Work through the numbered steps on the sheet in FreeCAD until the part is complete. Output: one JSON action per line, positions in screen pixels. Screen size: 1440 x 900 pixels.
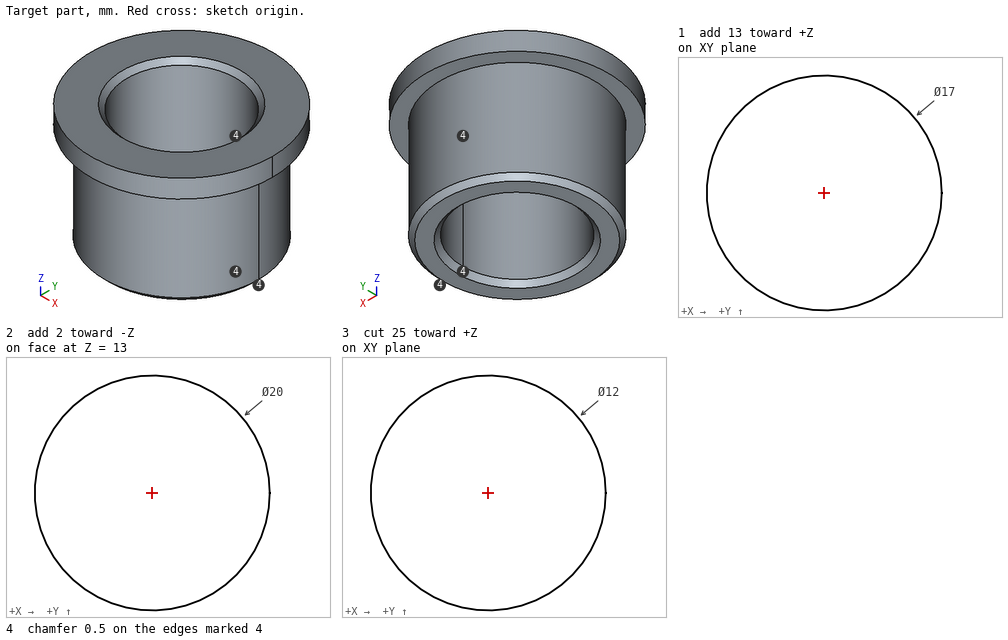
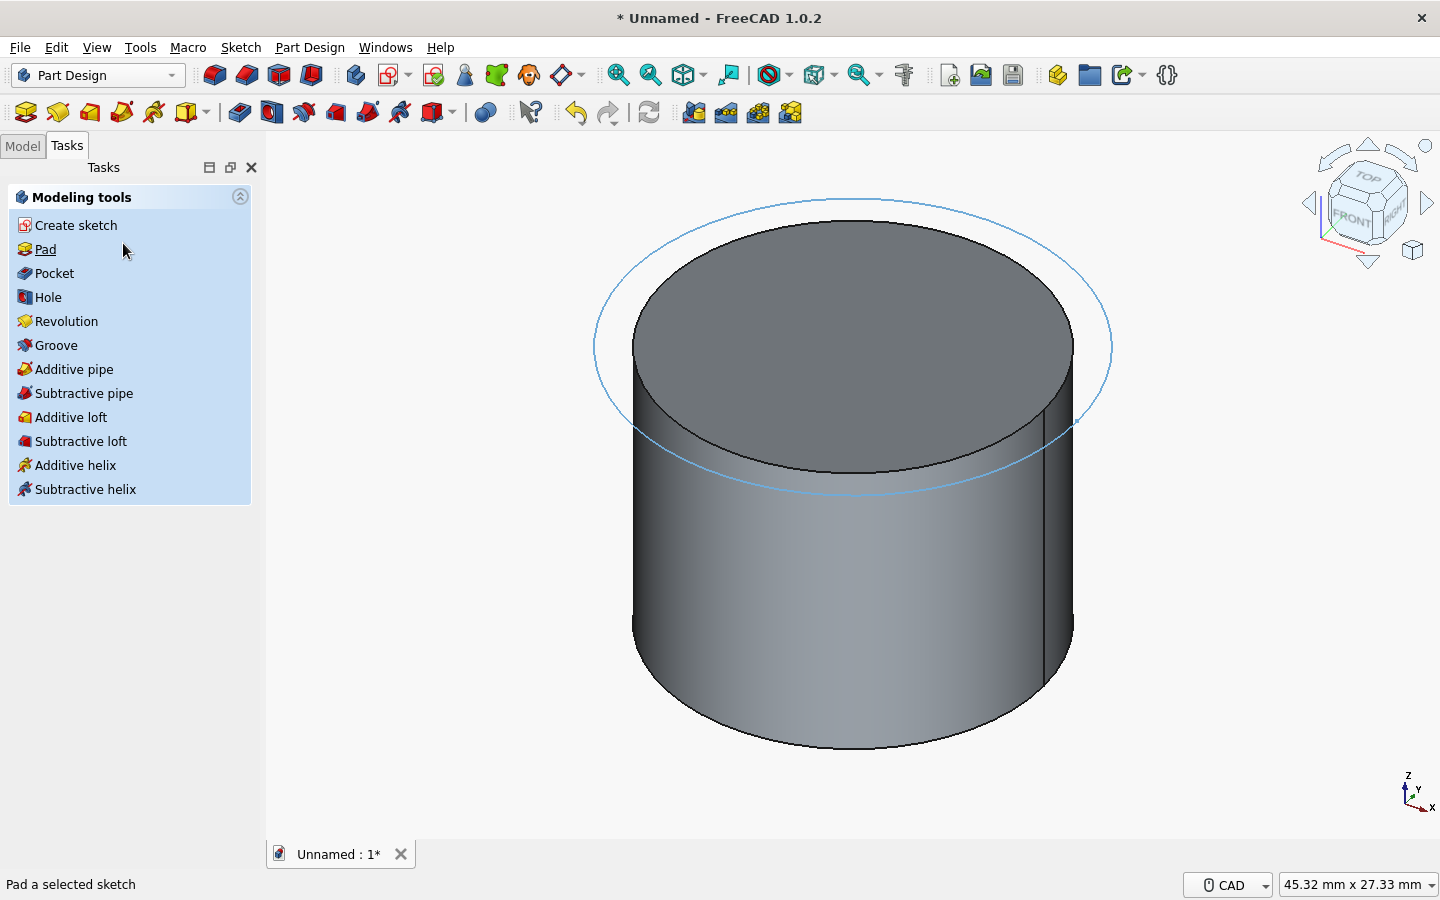
{"action": "left_click", "coordinate": [26, 112]}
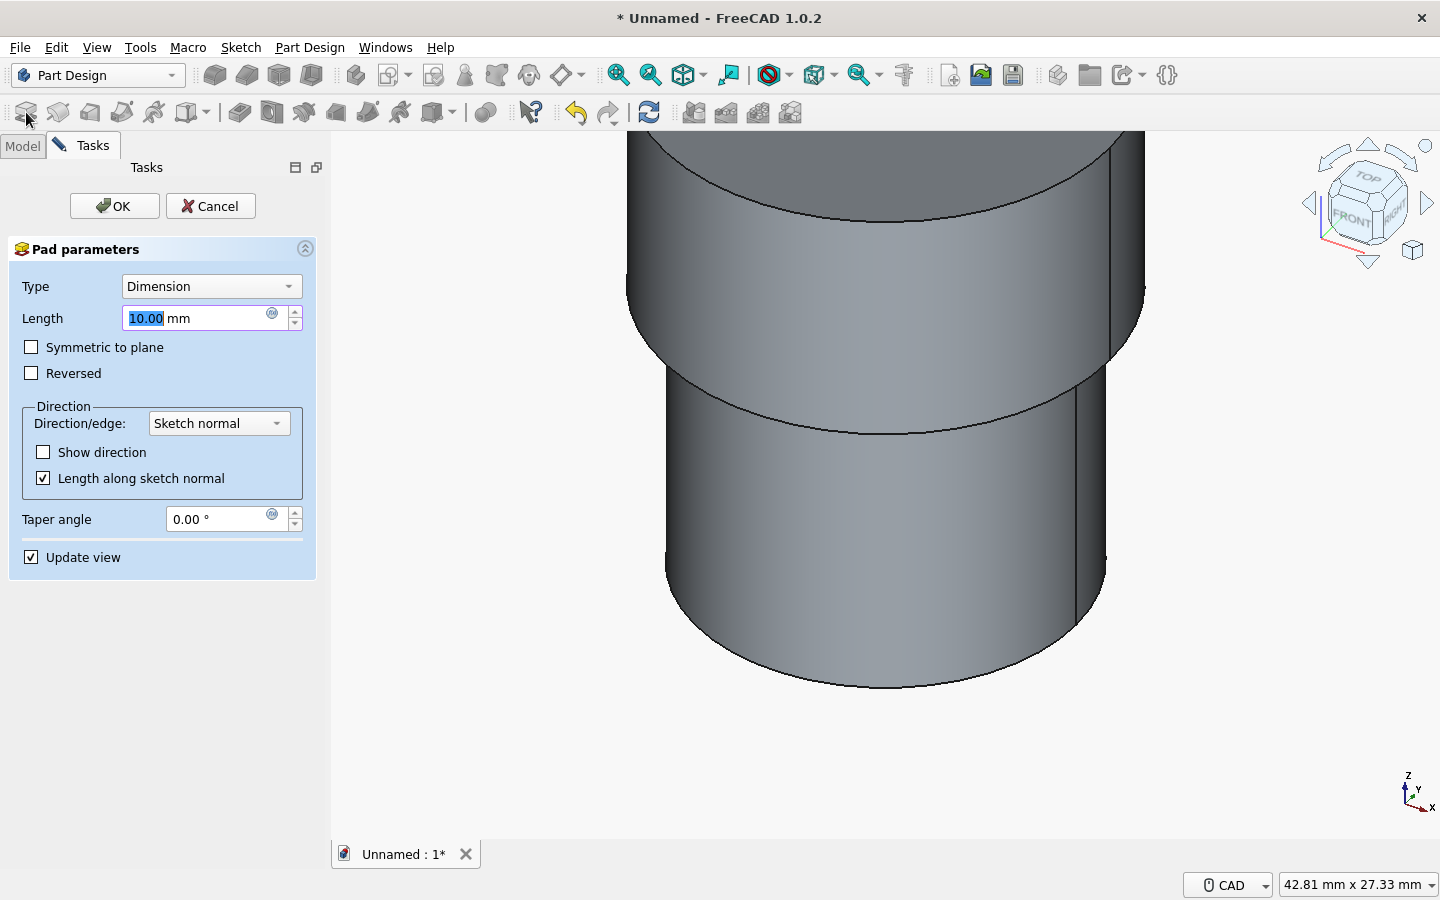
{"action": "type", "text": "2"}
{"action": "key", "text": "Tab"}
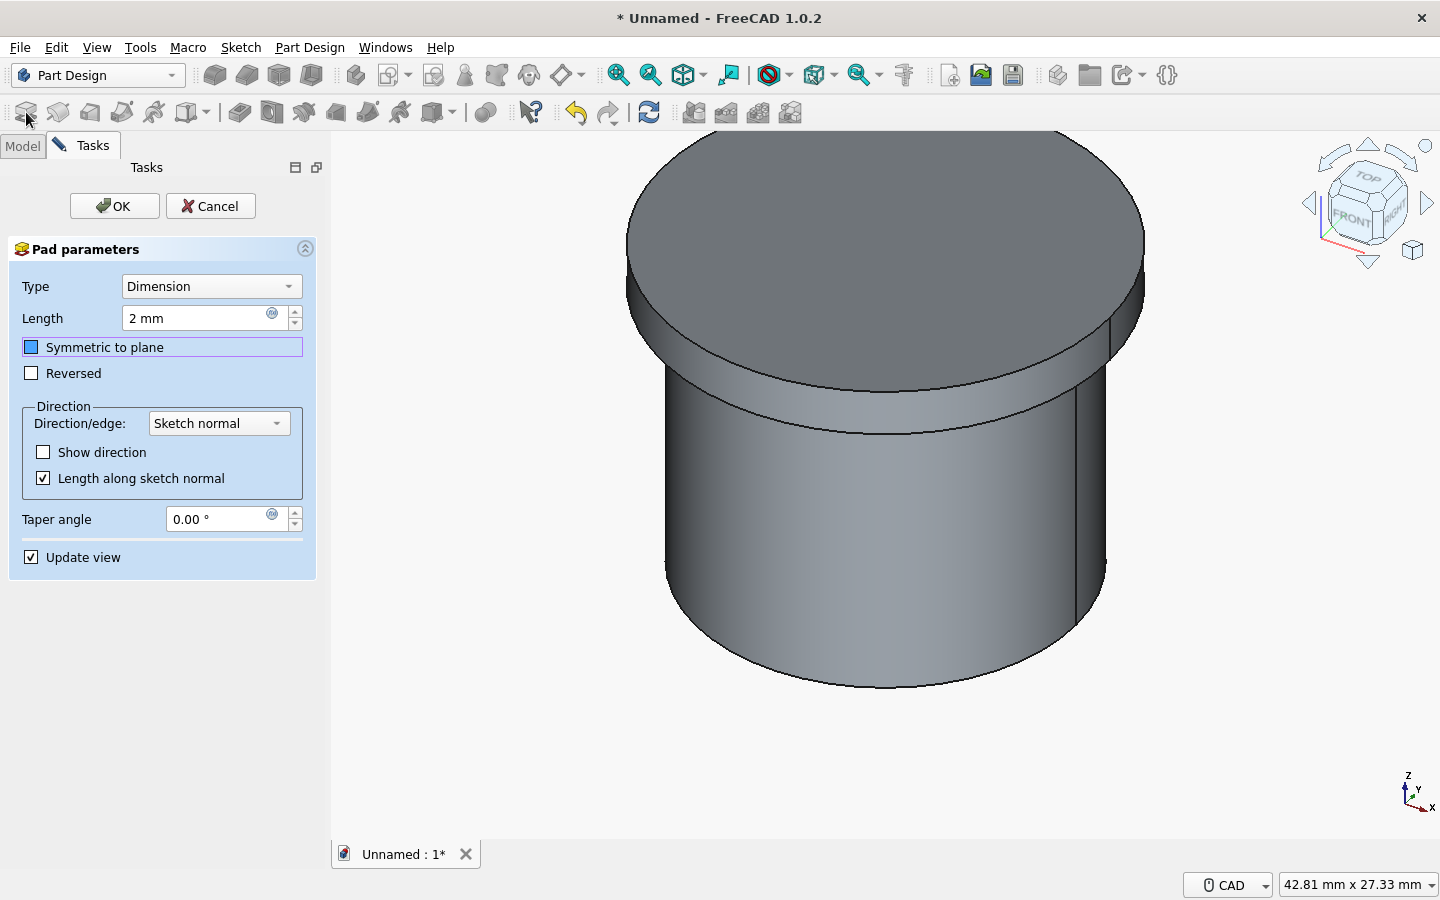
{"action": "left_click", "coordinate": [30, 373]}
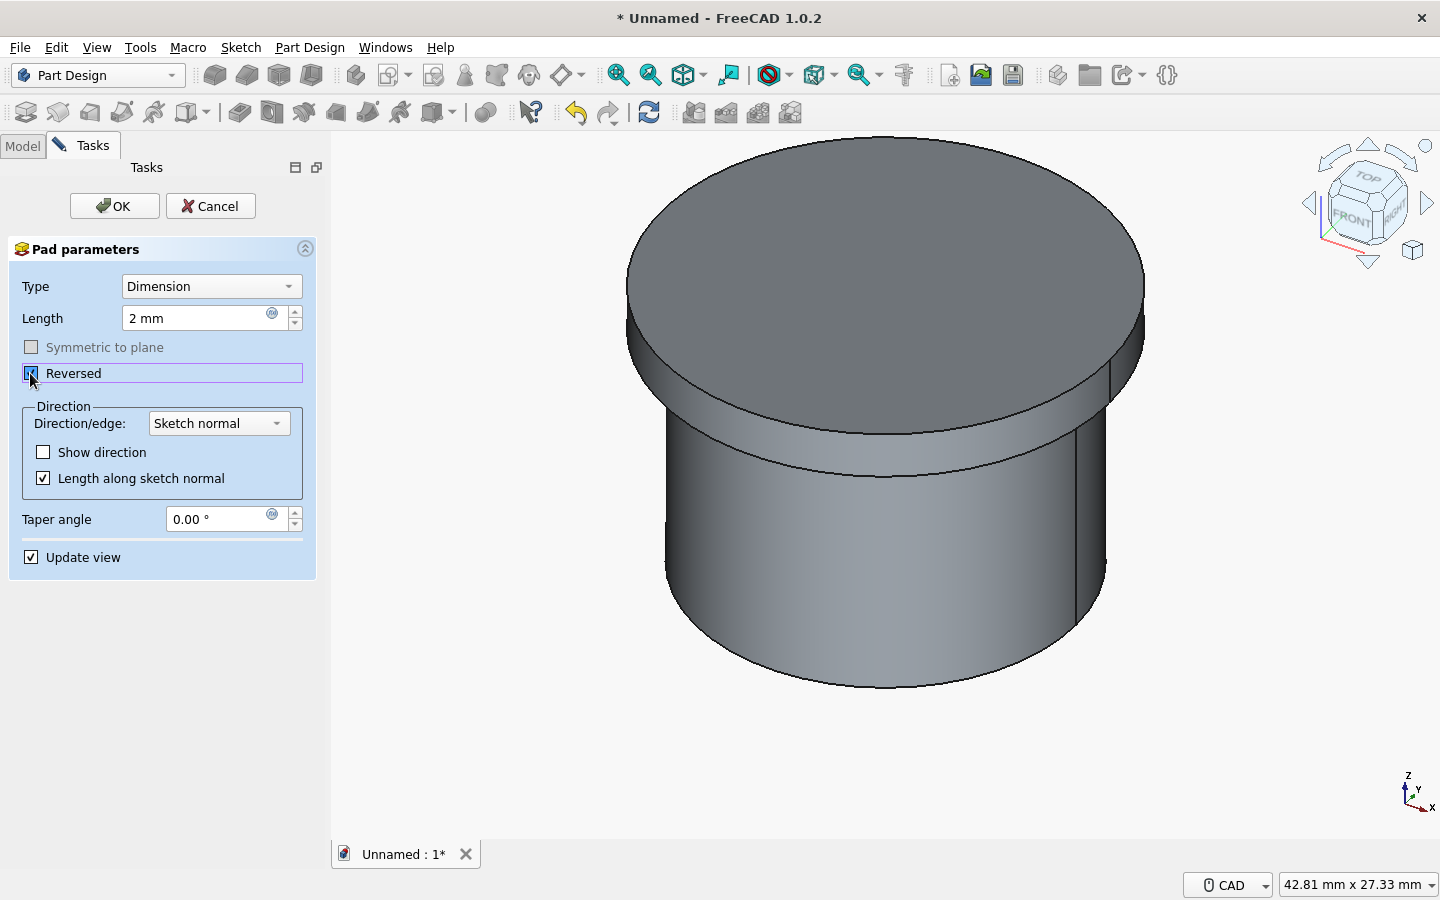
{"action": "left_click", "coordinate": [115, 206]}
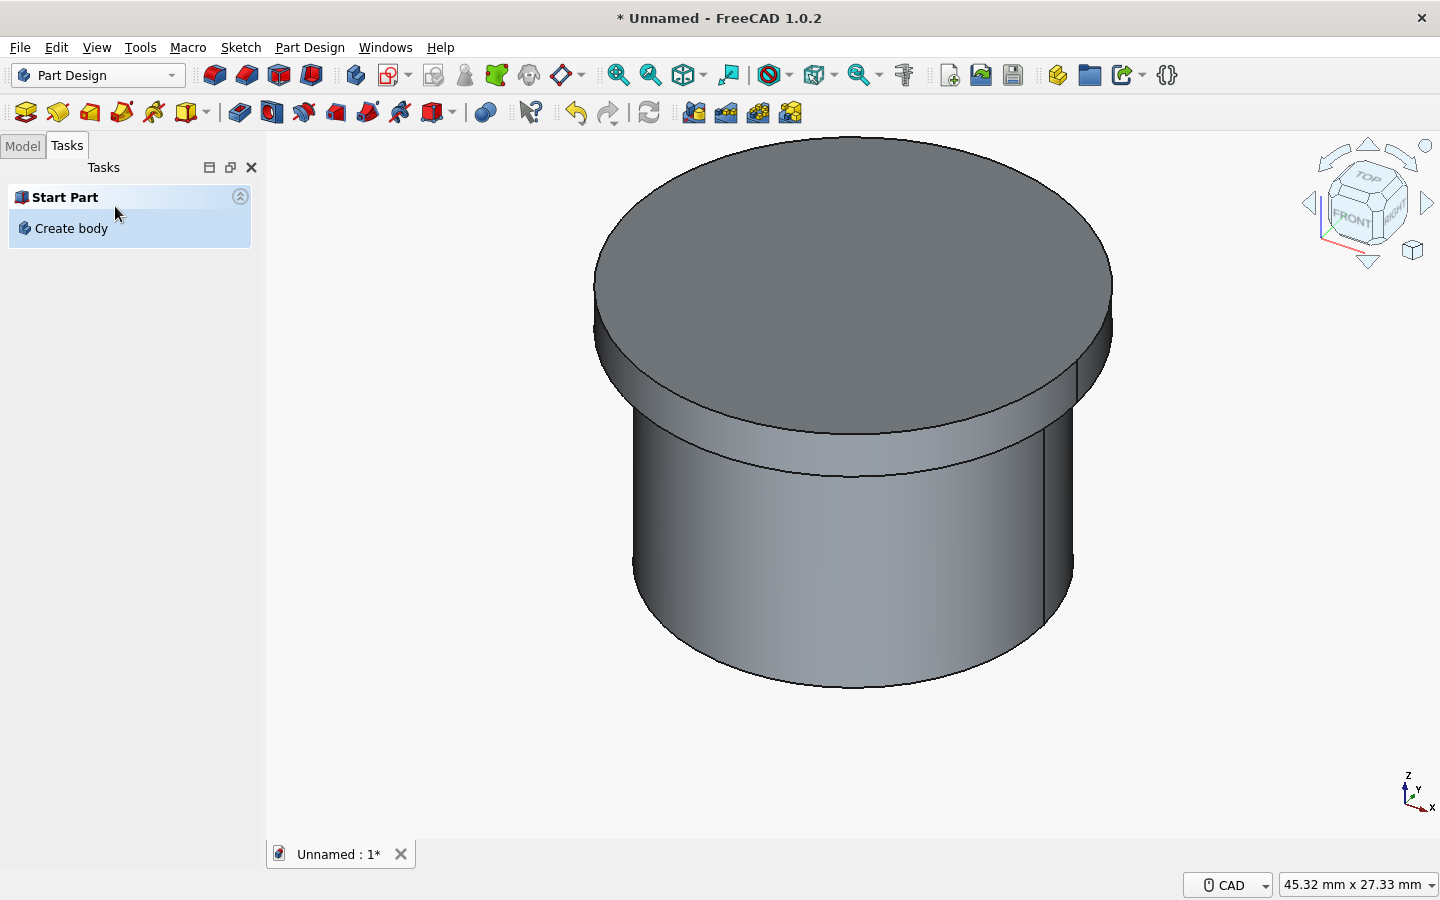
{"action": "key", "text": "v f"}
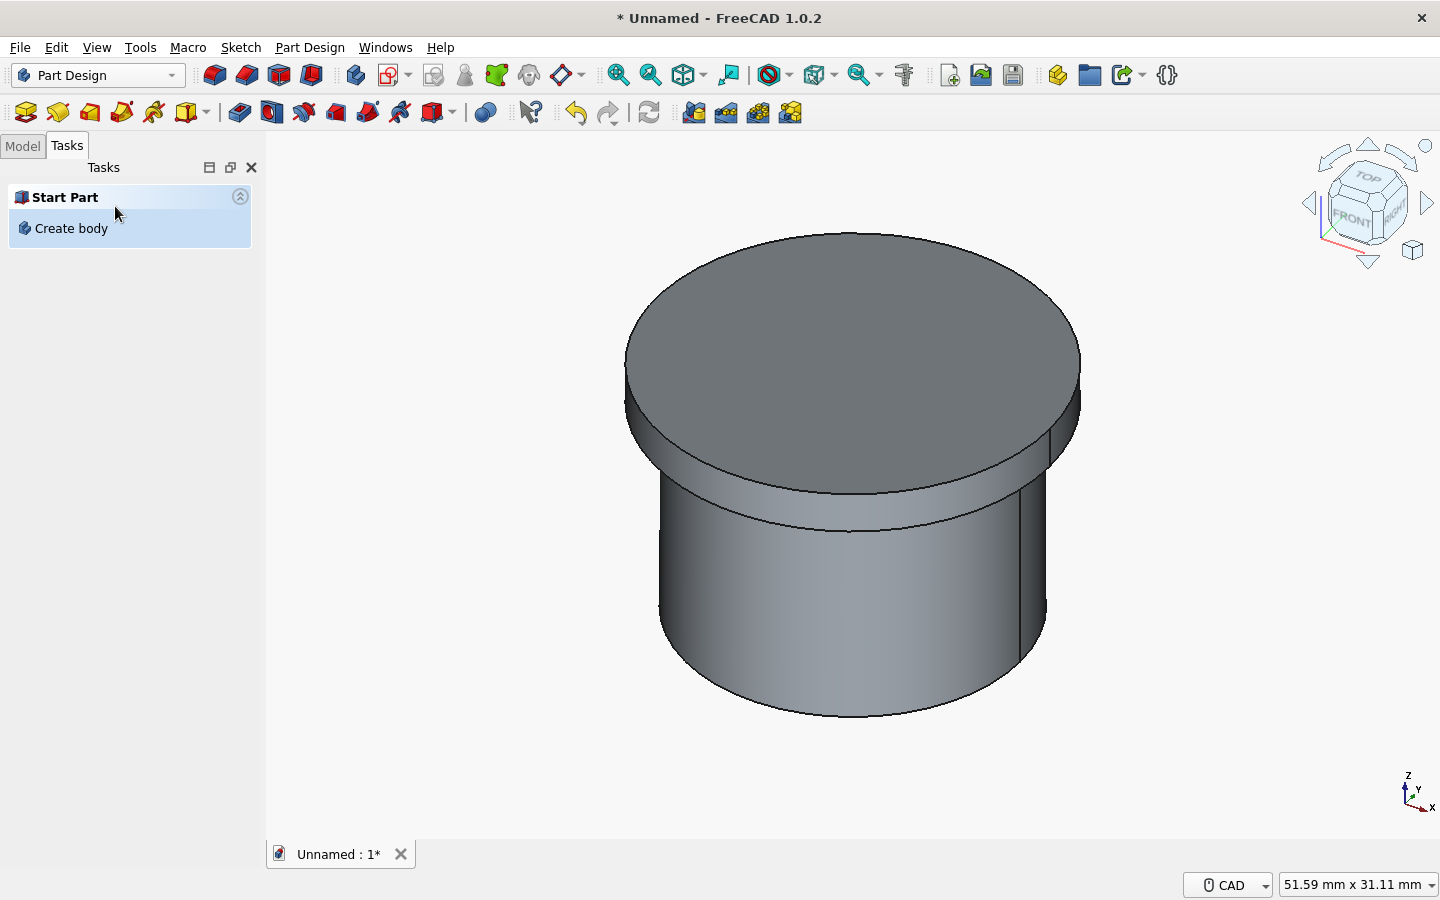
{"action": "left_click", "coordinate": [388, 76]}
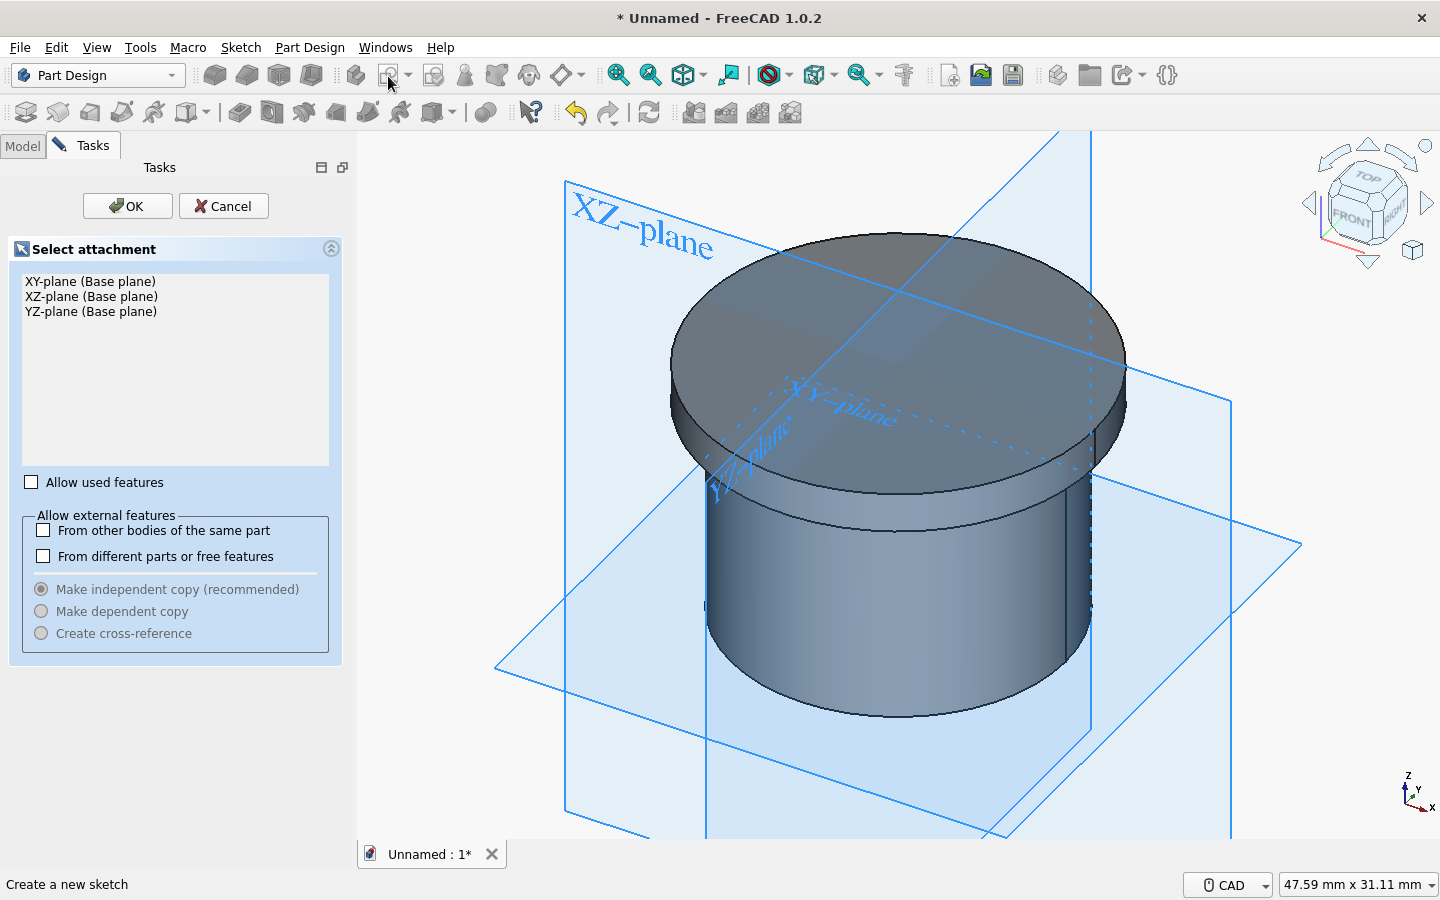
{"action": "left_click", "coordinate": [82, 282]}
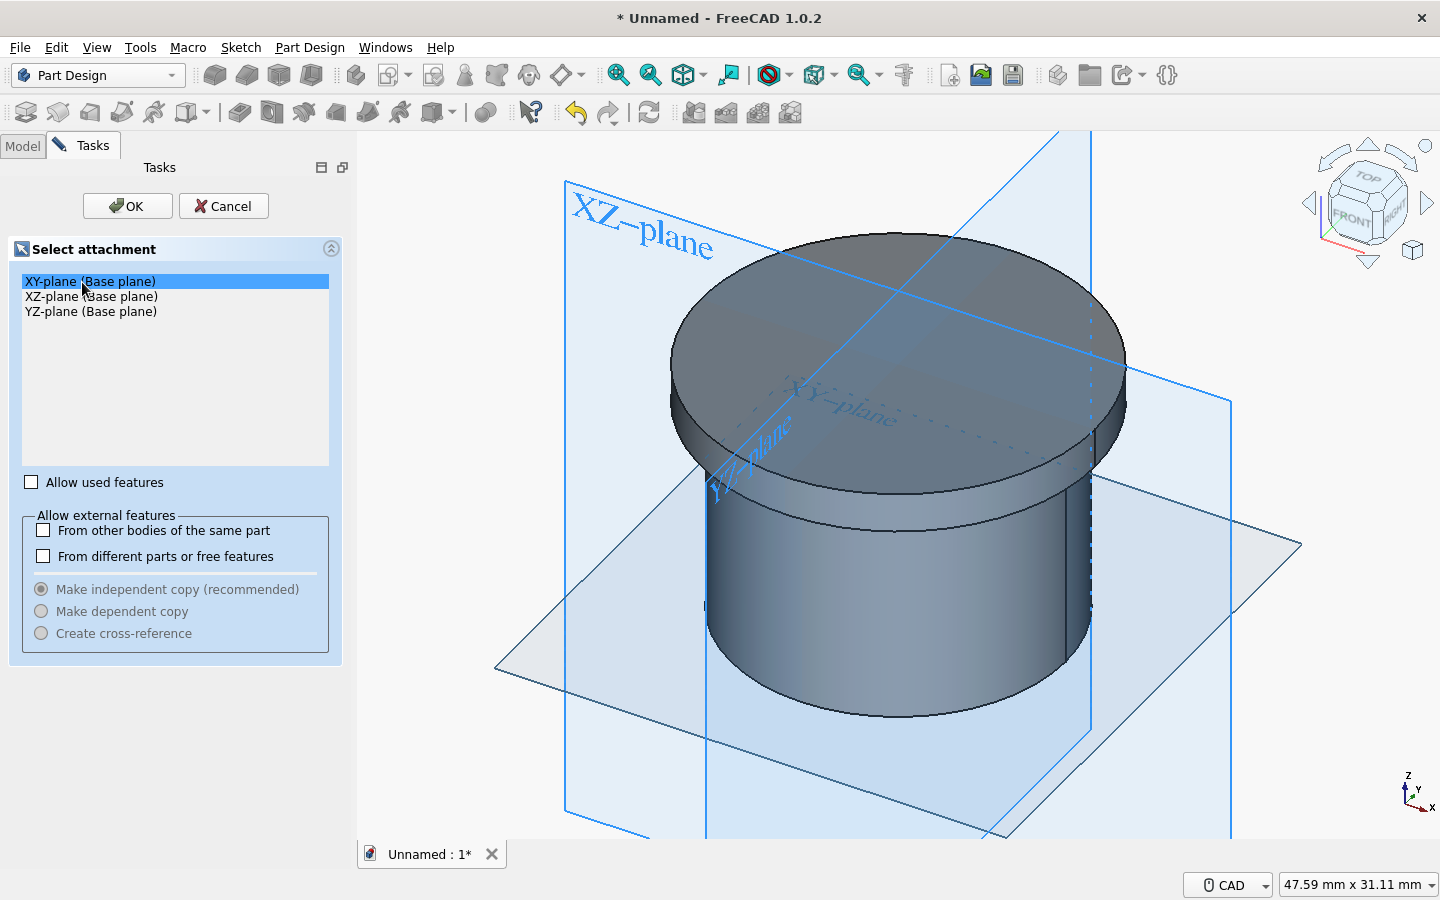
{"action": "left_click", "coordinate": [128, 206]}